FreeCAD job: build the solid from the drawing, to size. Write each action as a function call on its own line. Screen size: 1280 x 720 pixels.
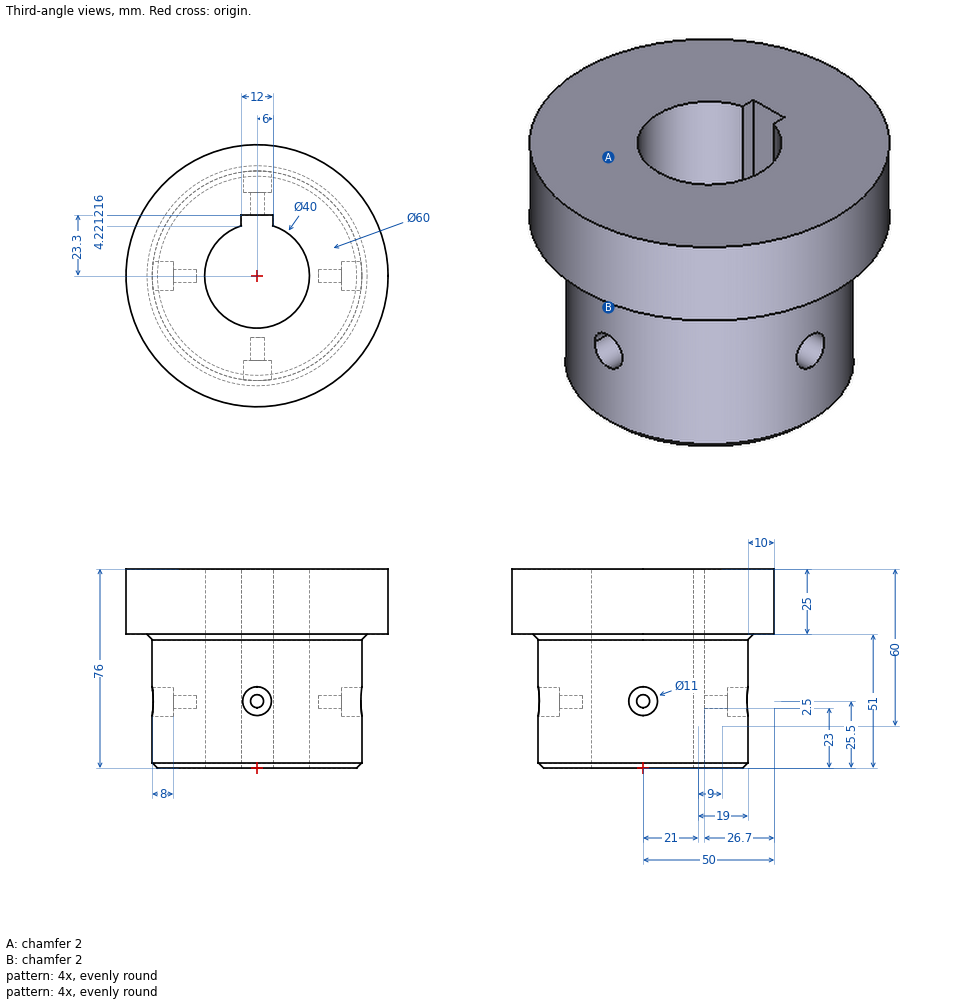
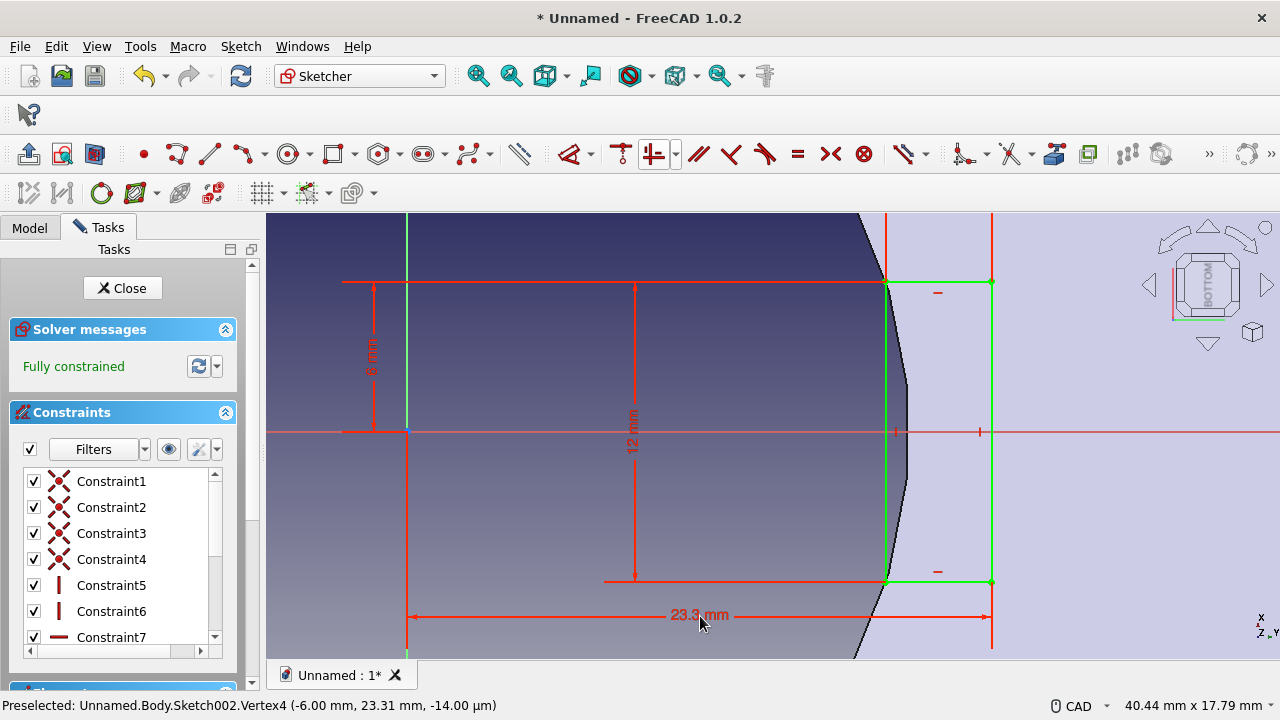
click(123, 288)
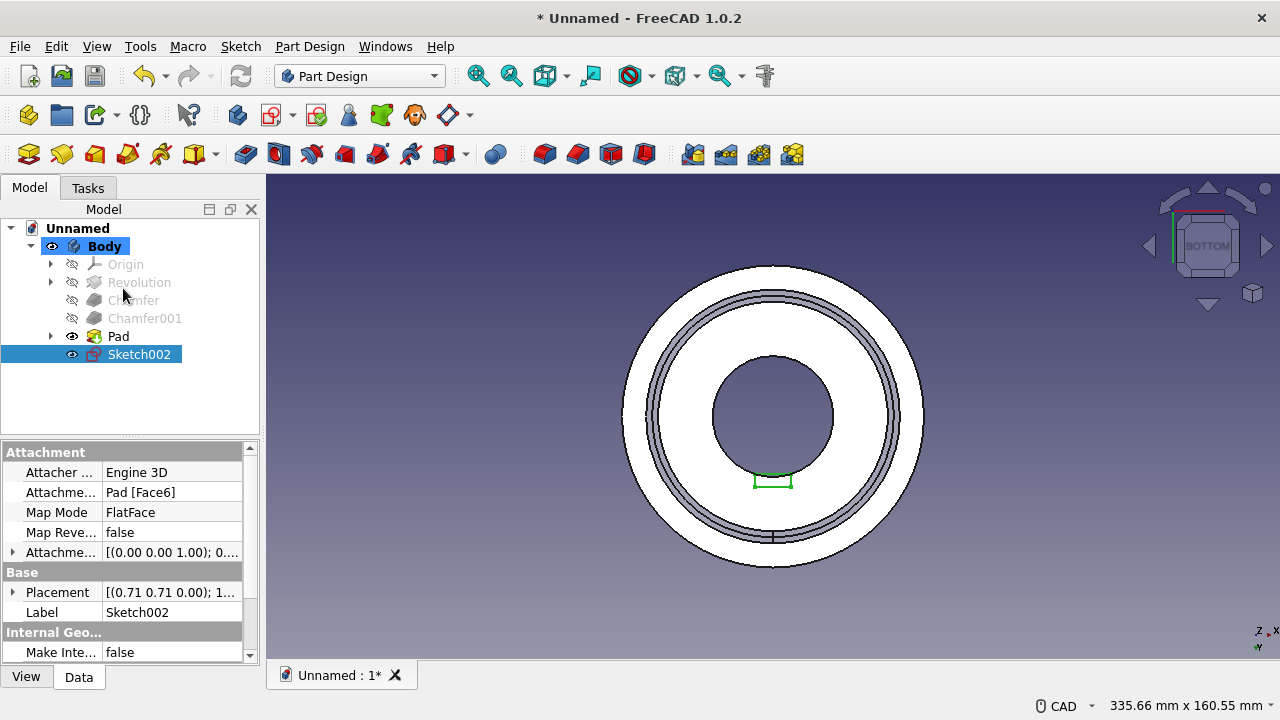
click(246, 154)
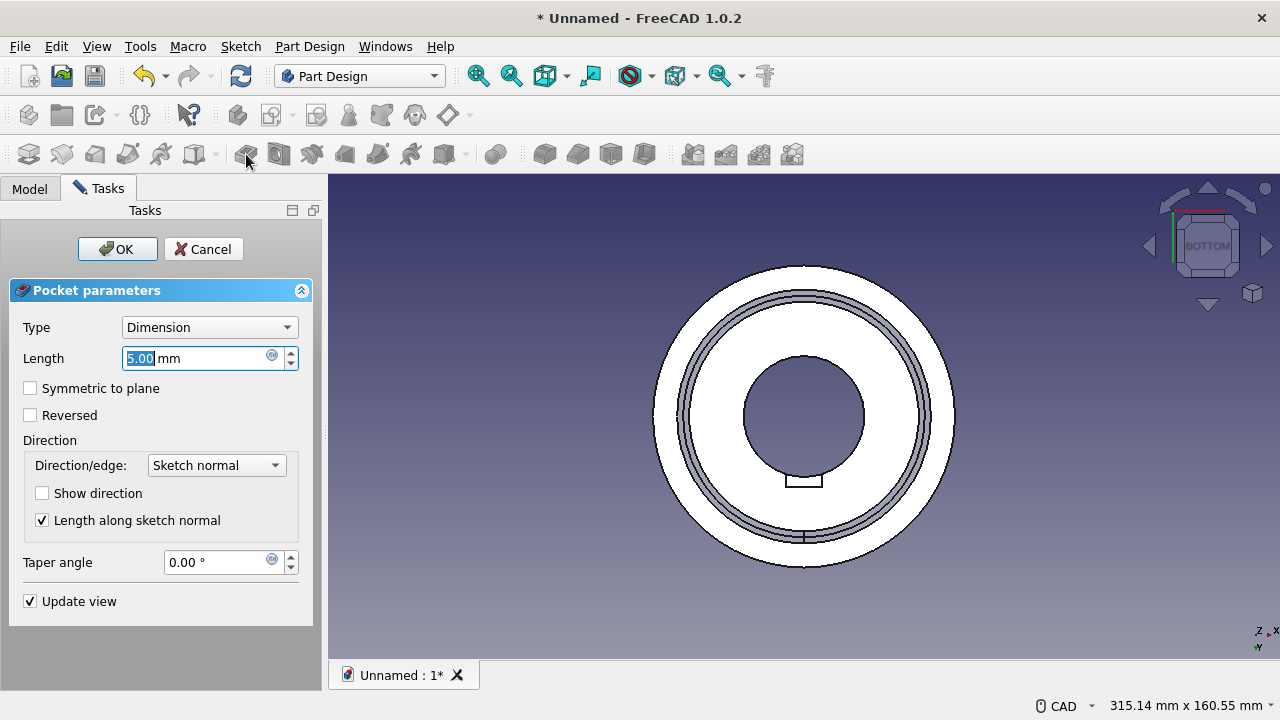
click(210, 328)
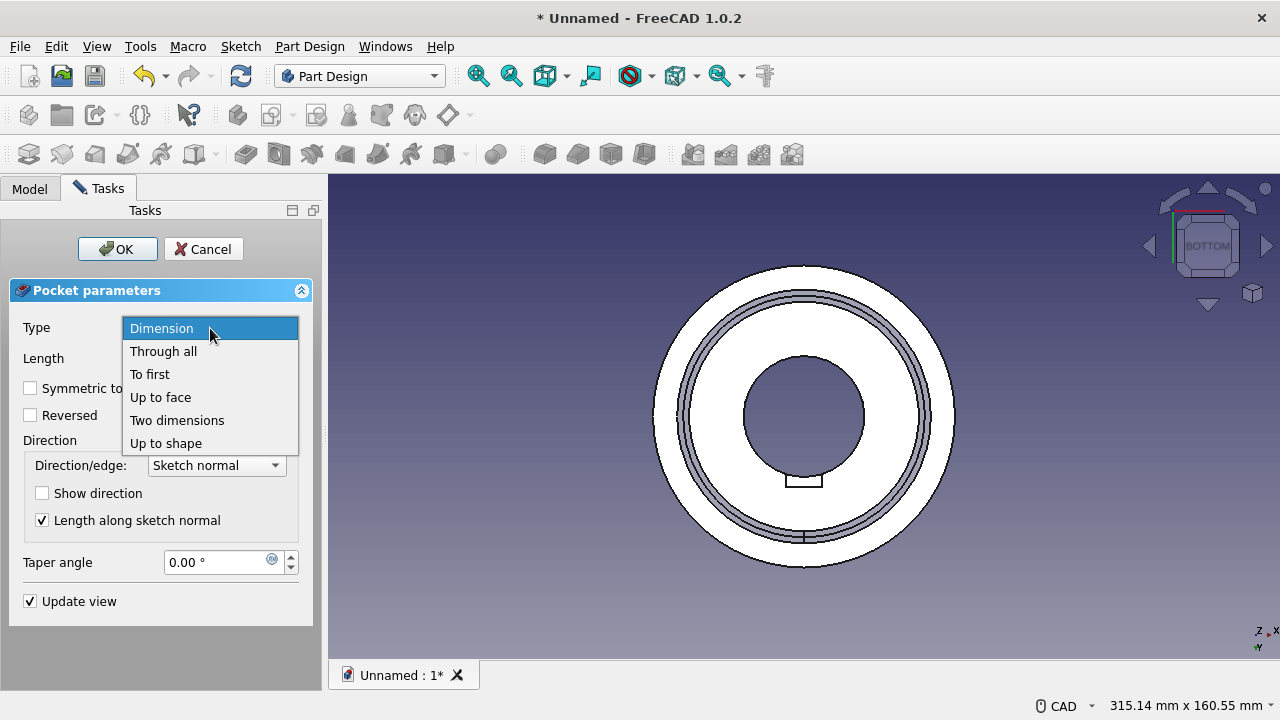
click(208, 352)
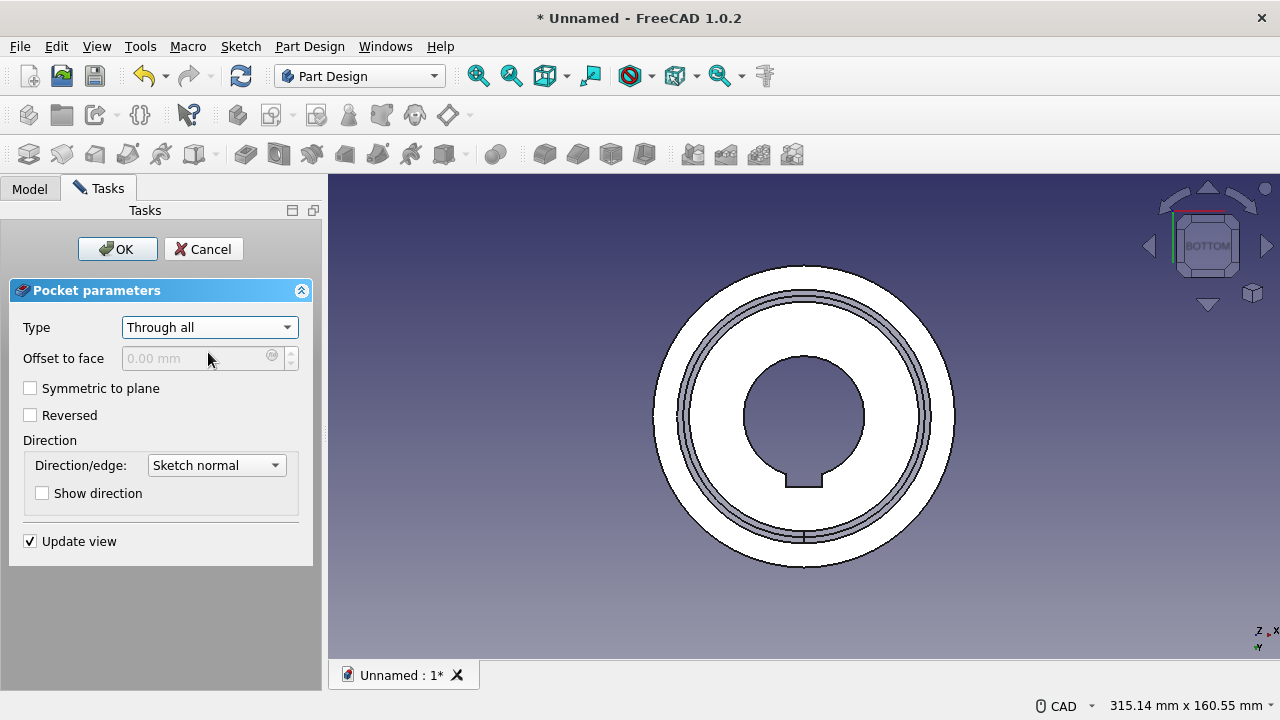
click(118, 249)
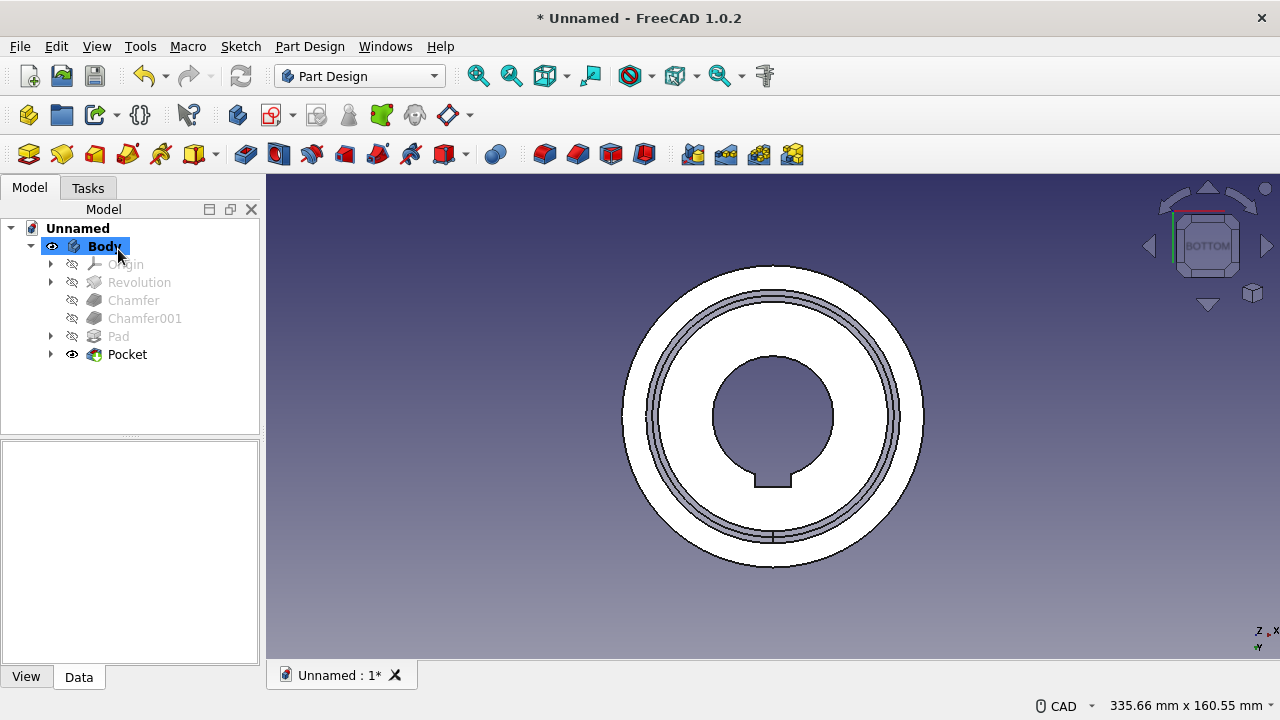
click(270, 116)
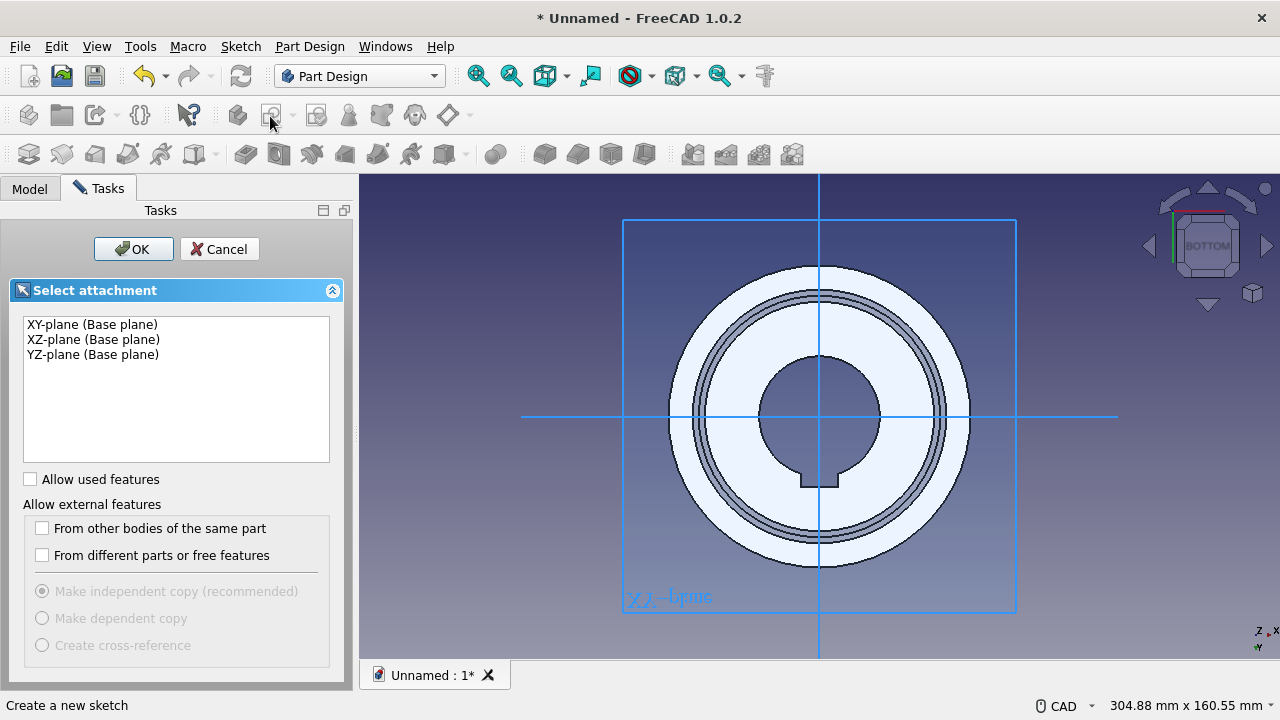
click(84, 354)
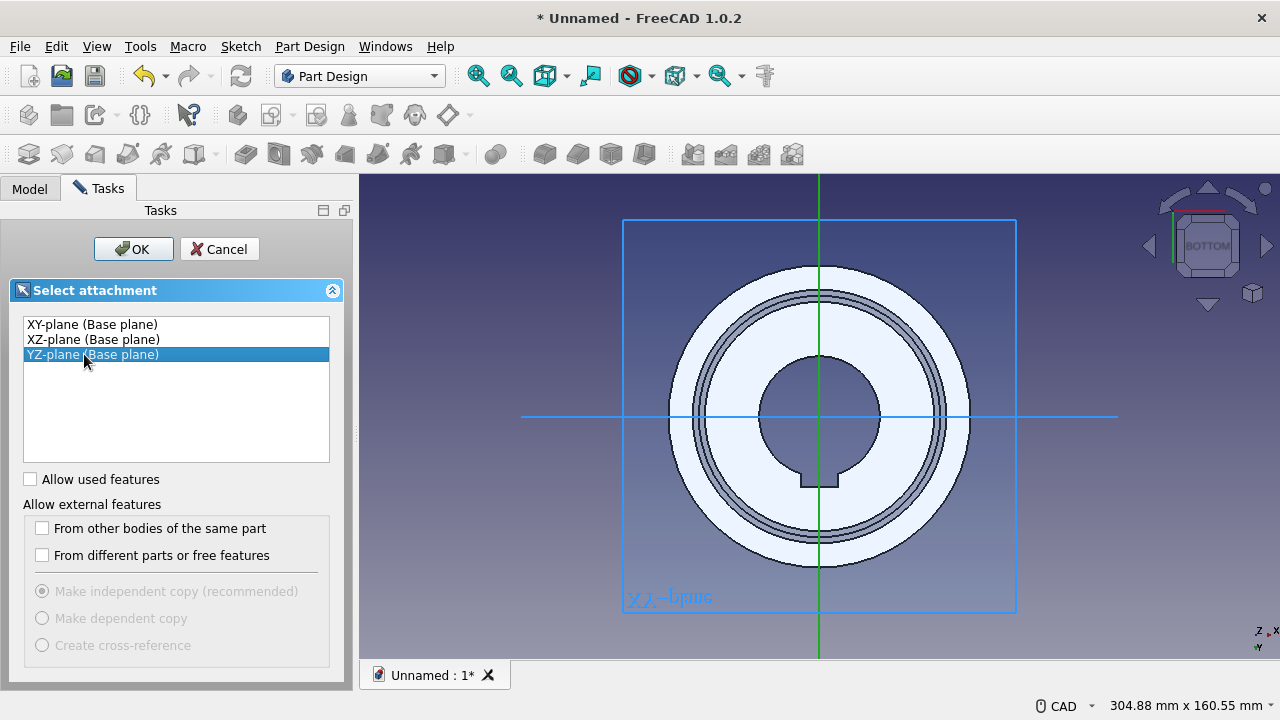
click(134, 249)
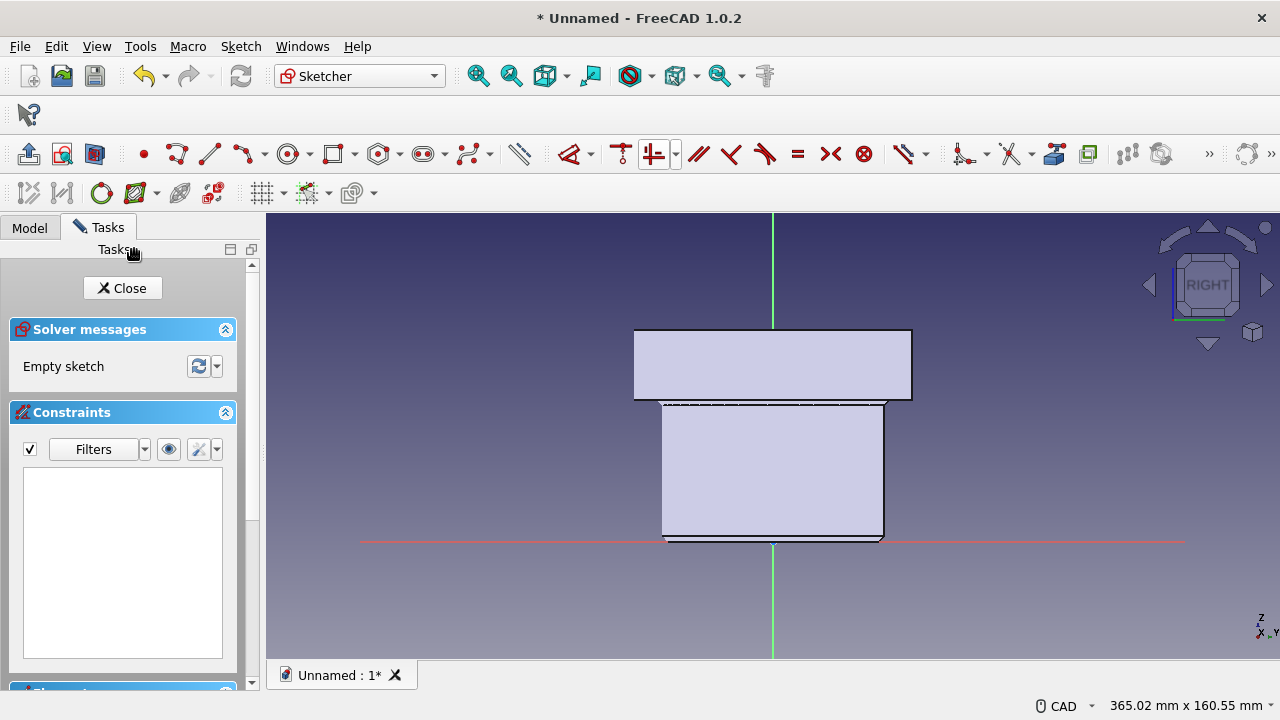
key(q)
key(s)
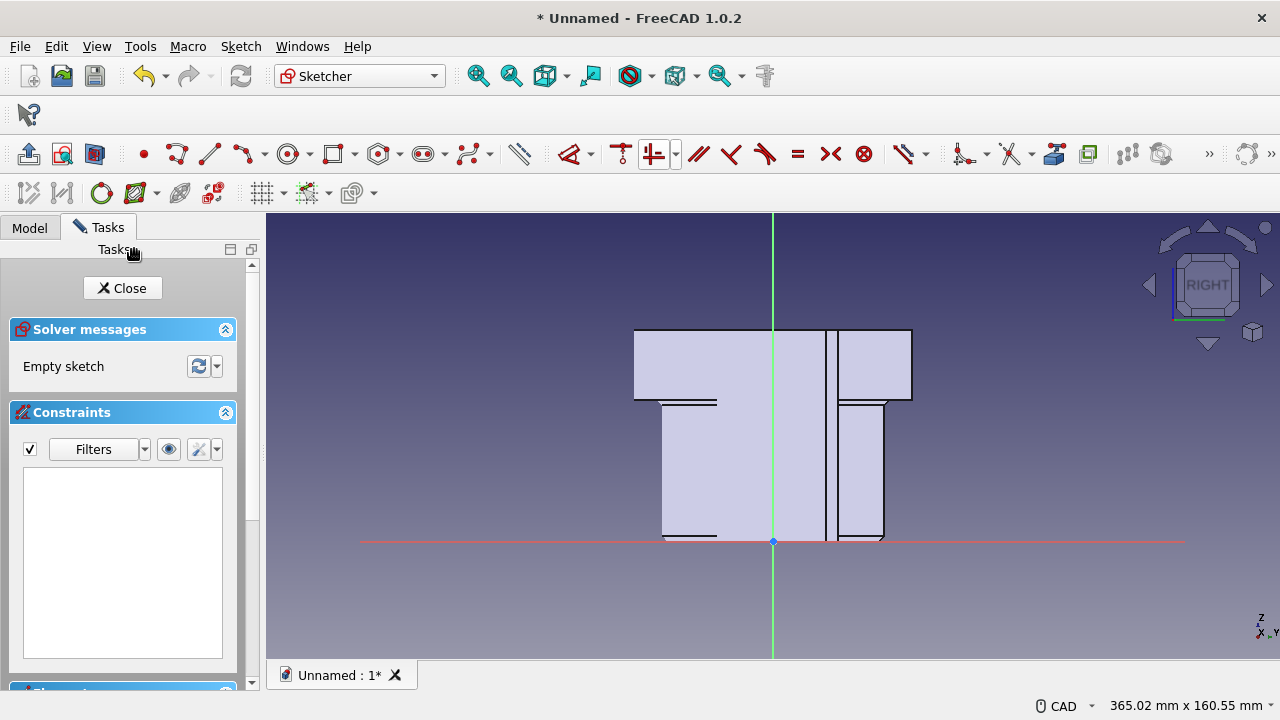
scroll(923, 536, up, 6)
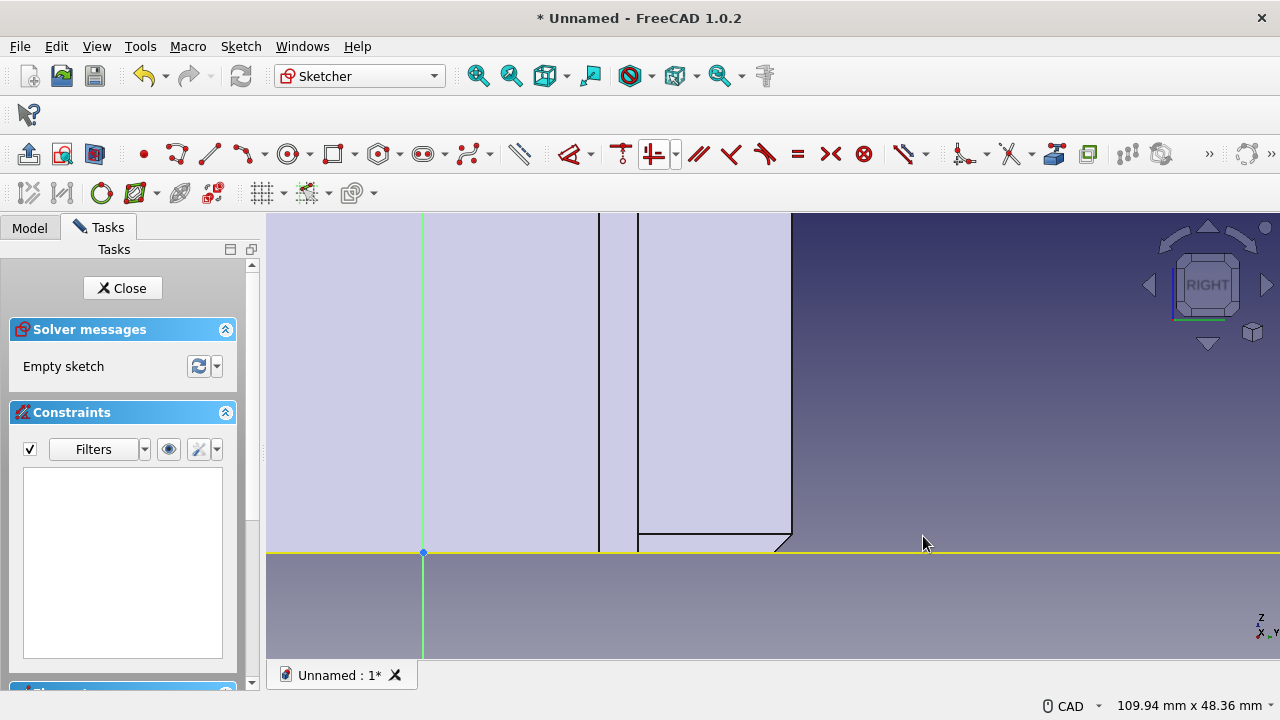
key(g)
key(r)